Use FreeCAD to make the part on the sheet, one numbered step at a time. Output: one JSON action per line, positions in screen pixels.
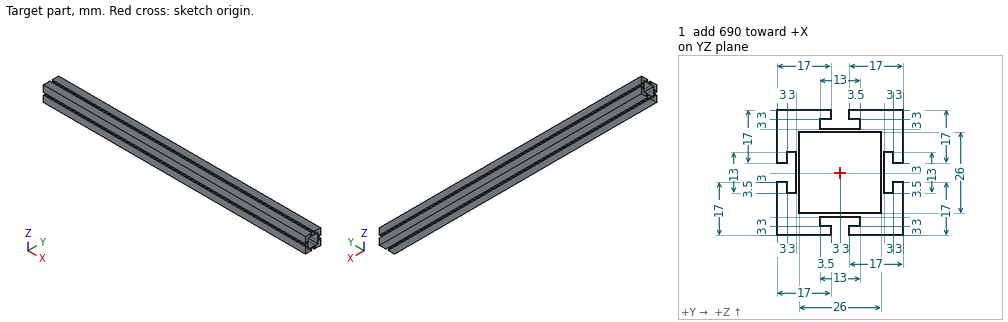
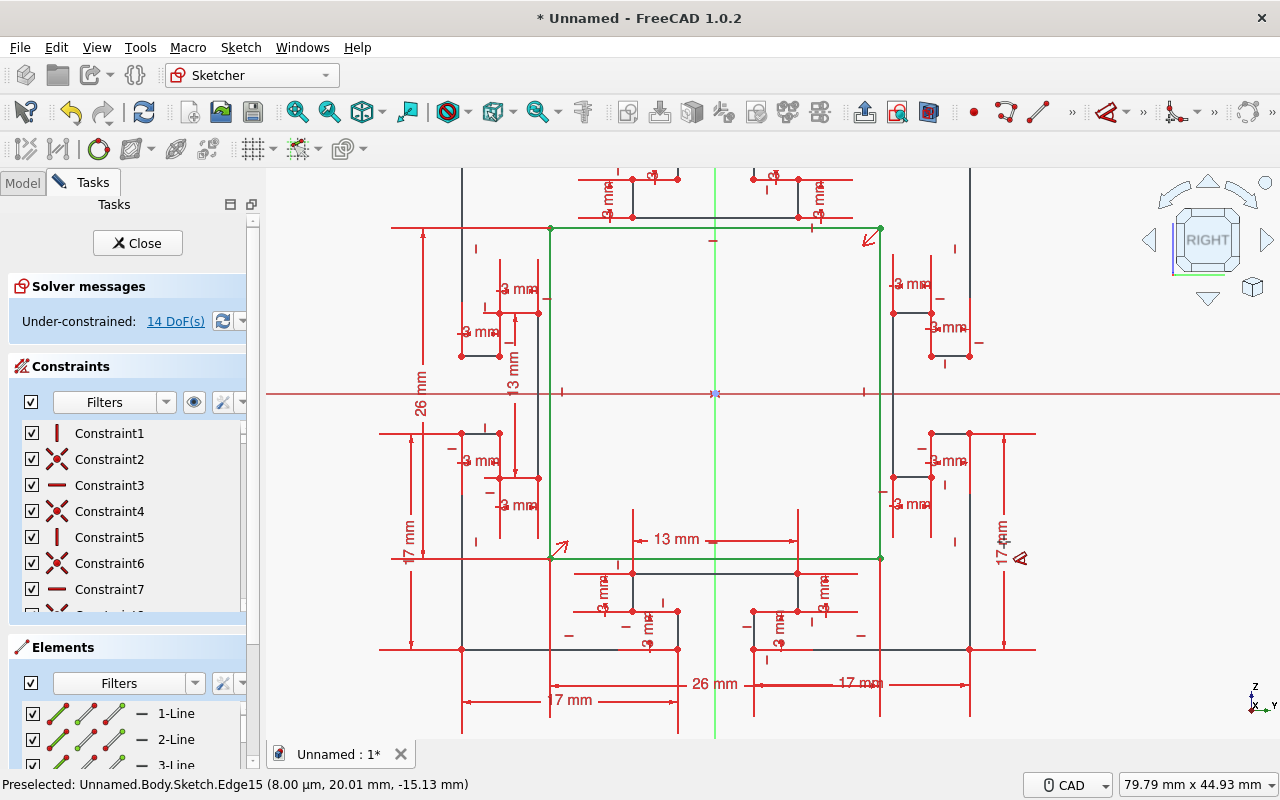
{"action": "left_click", "coordinate": [893, 428]}
{"action": "left_click", "coordinate": [859, 357]}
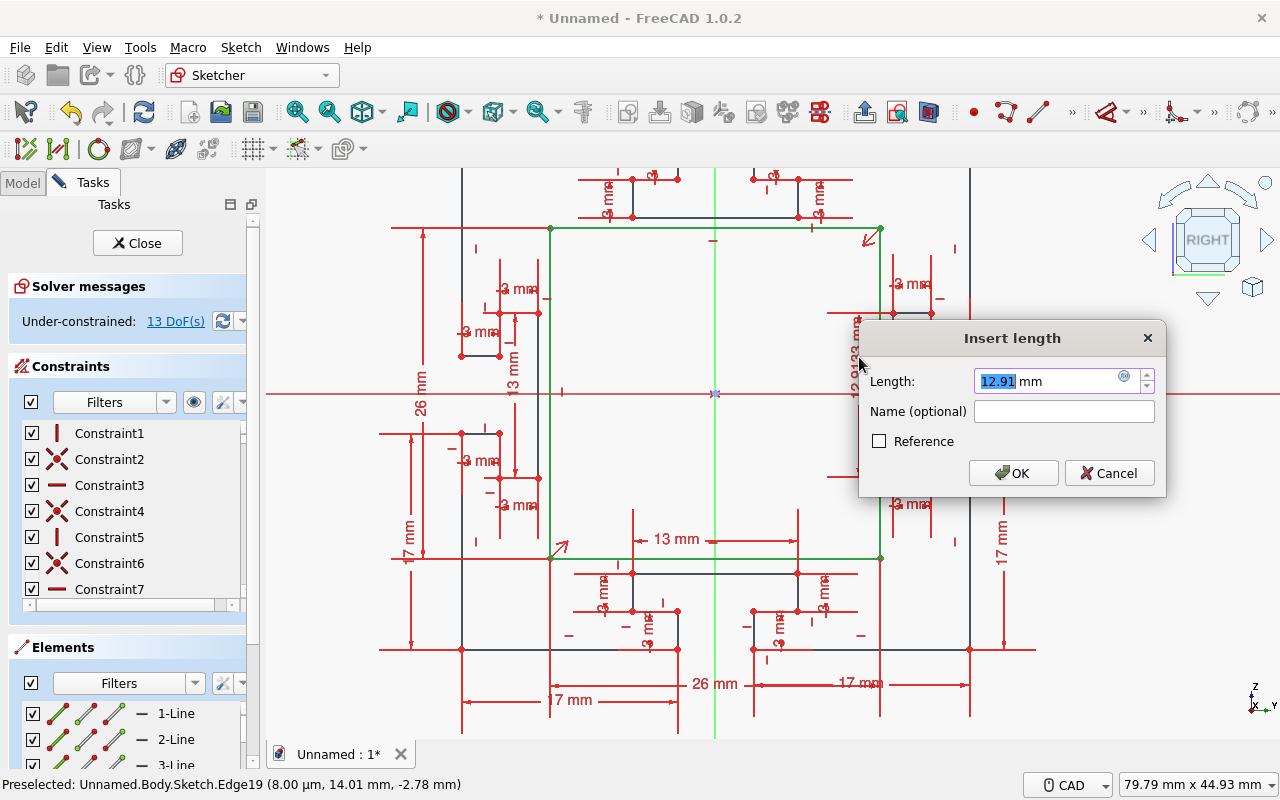
{"action": "type", "text": "13"}
{"action": "key", "text": "Return"}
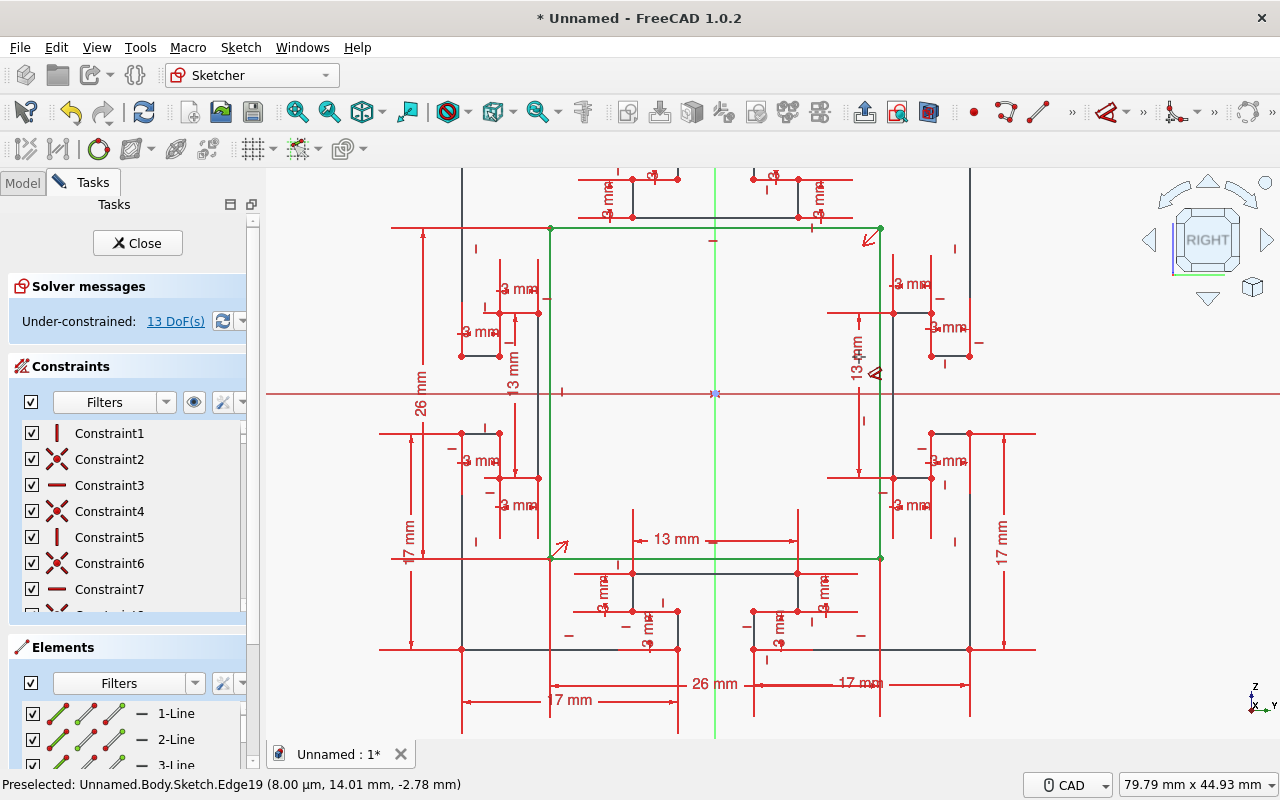
{"action": "left_click", "coordinate": [970, 292]}
{"action": "left_click", "coordinate": [1004, 276]}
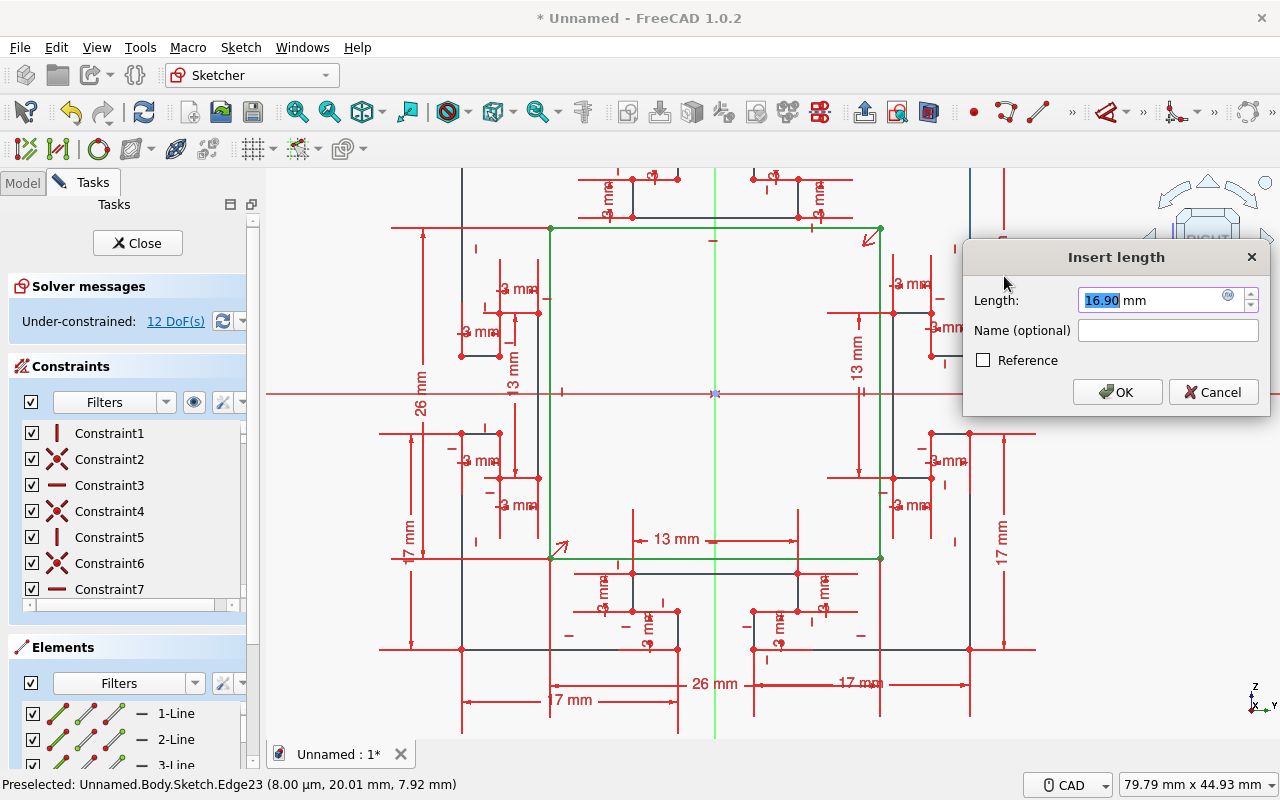
{"action": "type", "text": "17"}
{"action": "key", "text": "Return"}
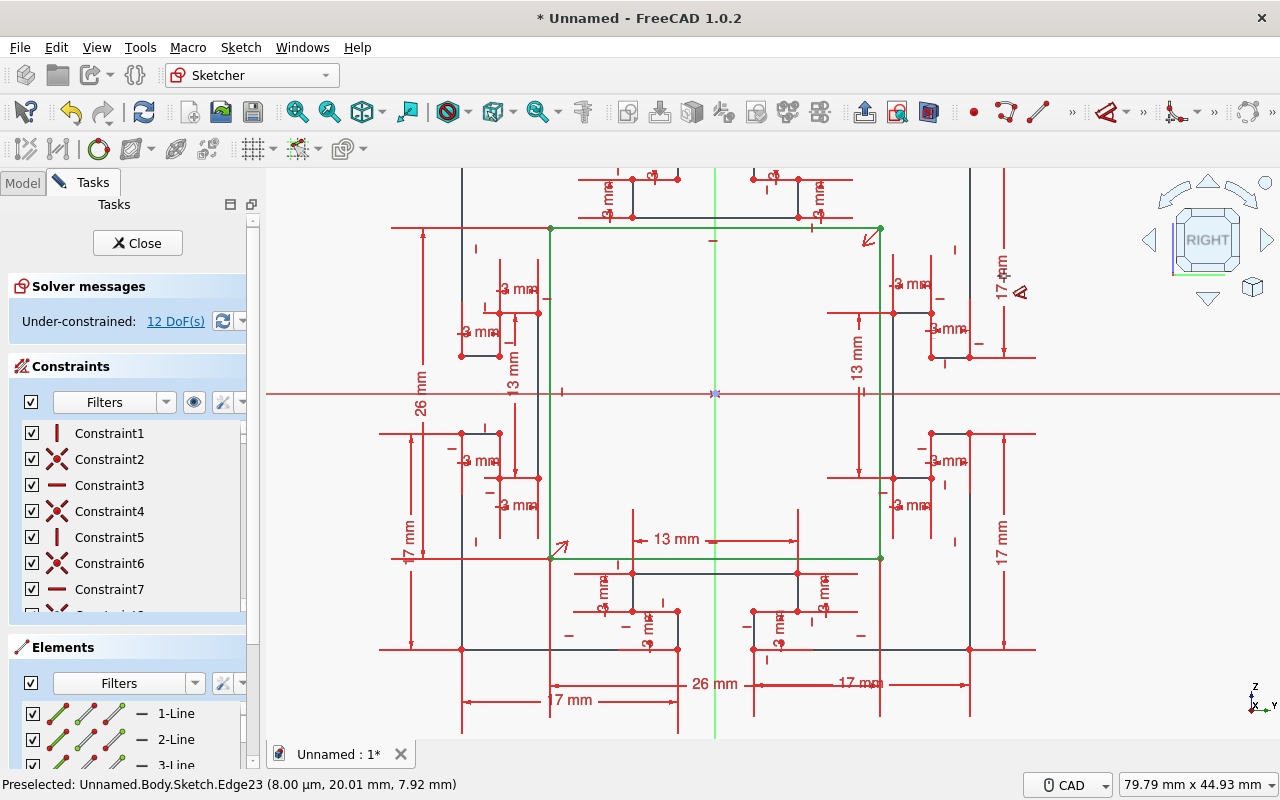
{"action": "scroll", "coordinate": [683, 575], "scroll_direction": "down", "scroll_amount": 2}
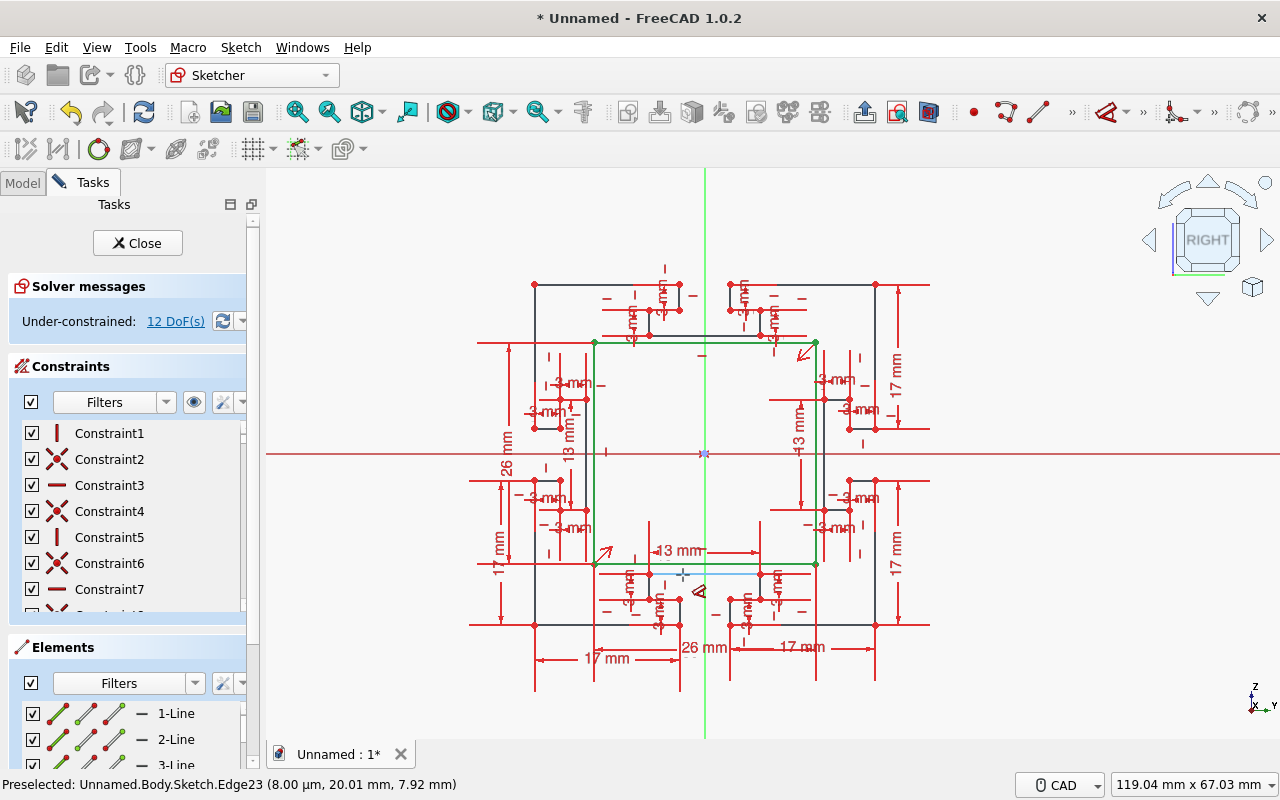
{"action": "left_click", "coordinate": [832, 285]}
{"action": "left_click", "coordinate": [803, 251]}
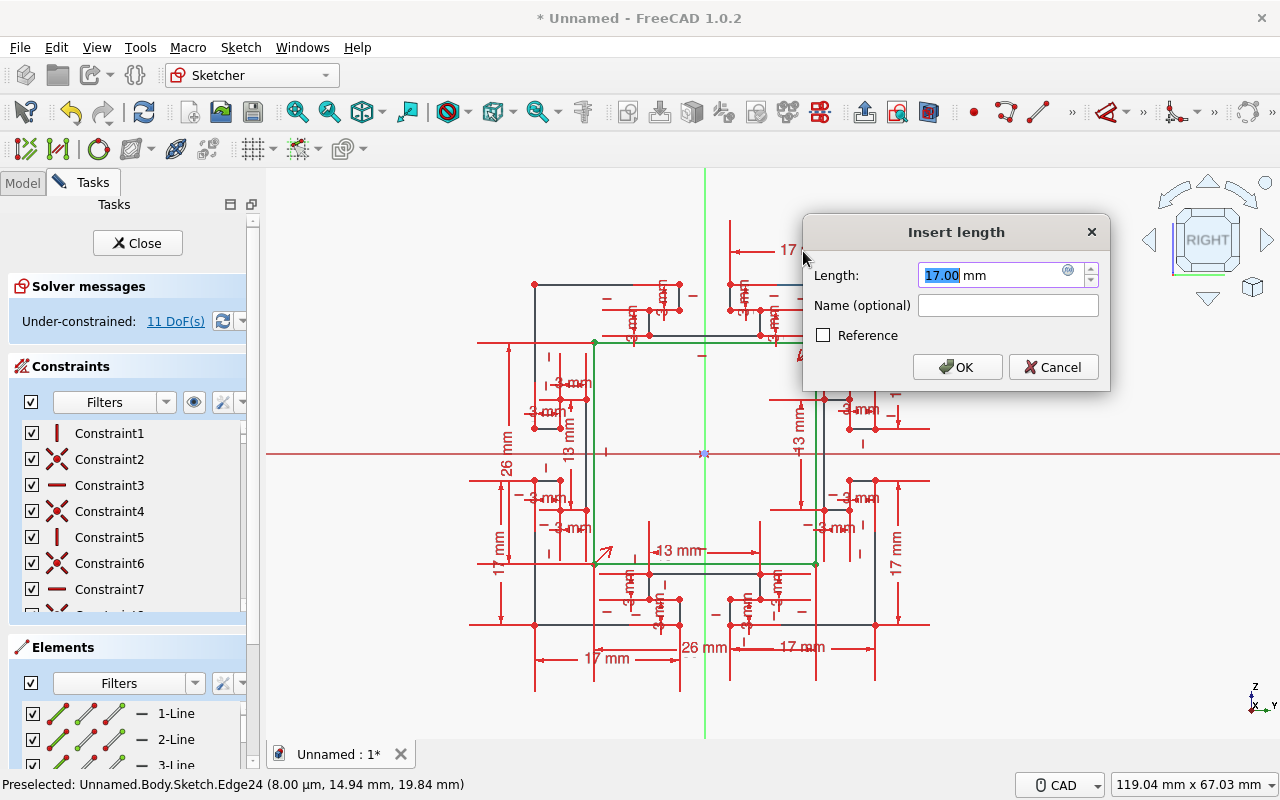
{"action": "type", "text": "17"}
{"action": "key", "text": "Return"}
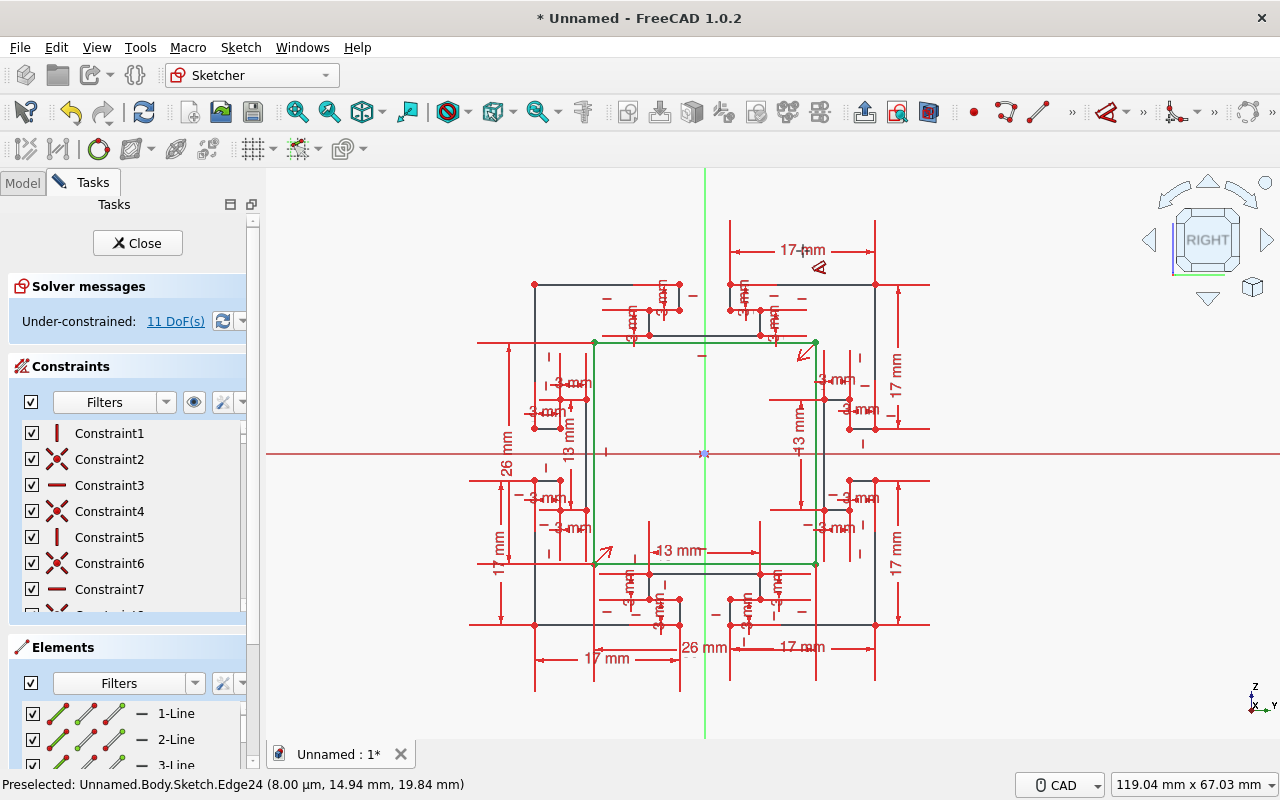
{"action": "scroll", "coordinate": [727, 336], "scroll_direction": "up", "scroll_amount": 4}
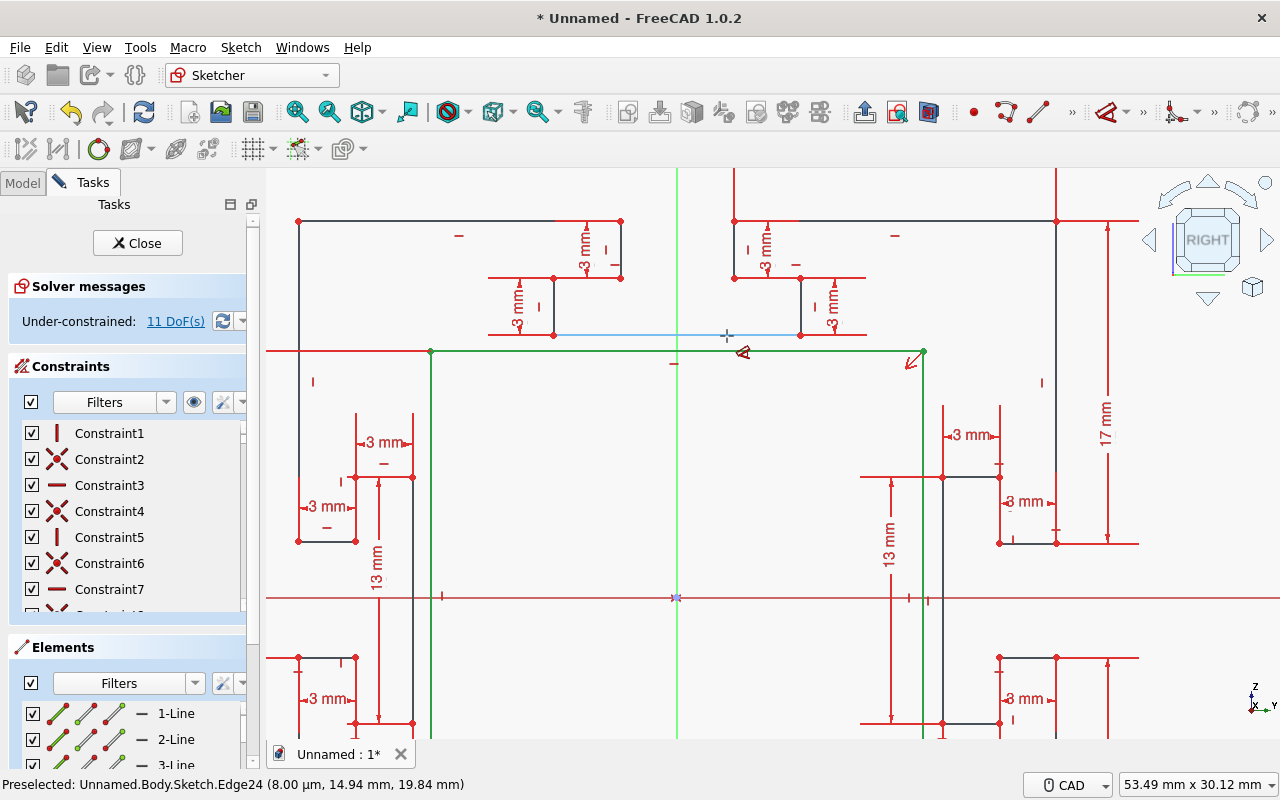
{"action": "left_click", "coordinate": [727, 335]}
{"action": "left_click", "coordinate": [621, 301]}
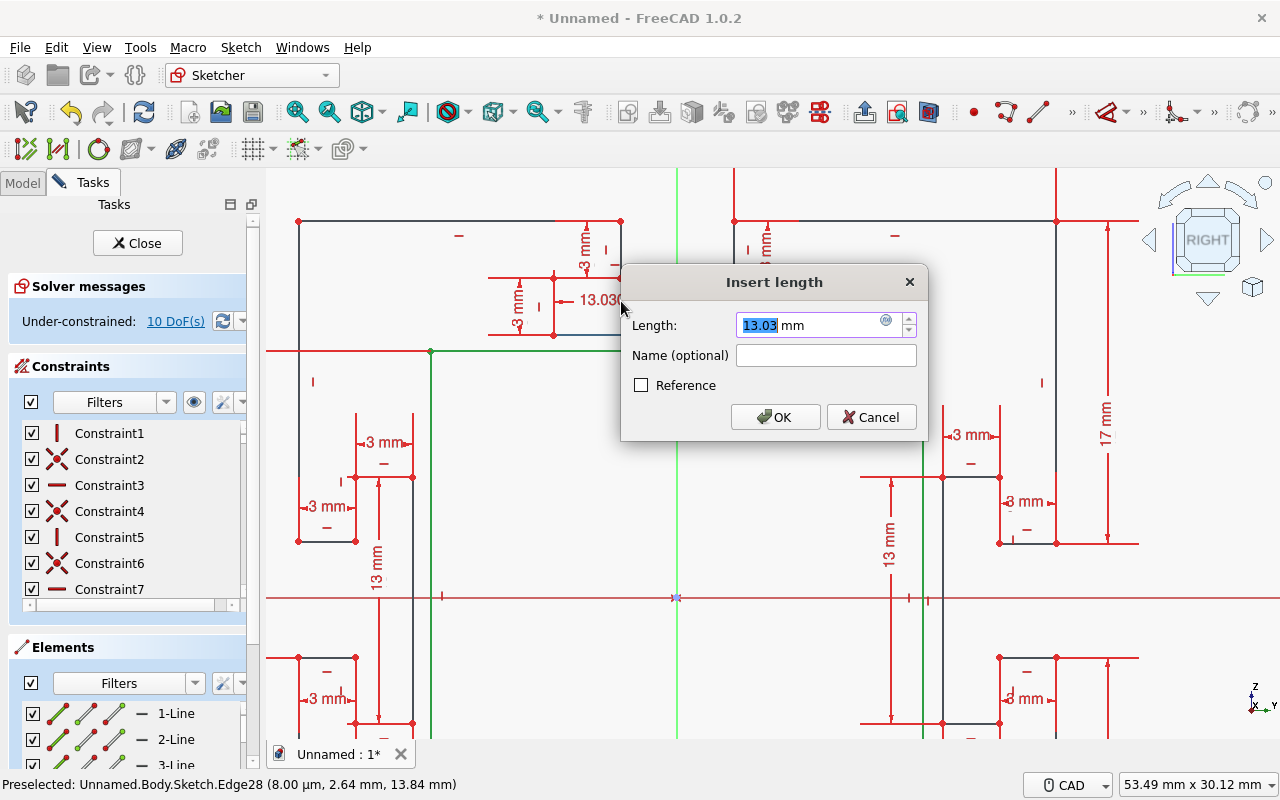
{"action": "type", "text": "13"}
{"action": "key", "text": "Return"}